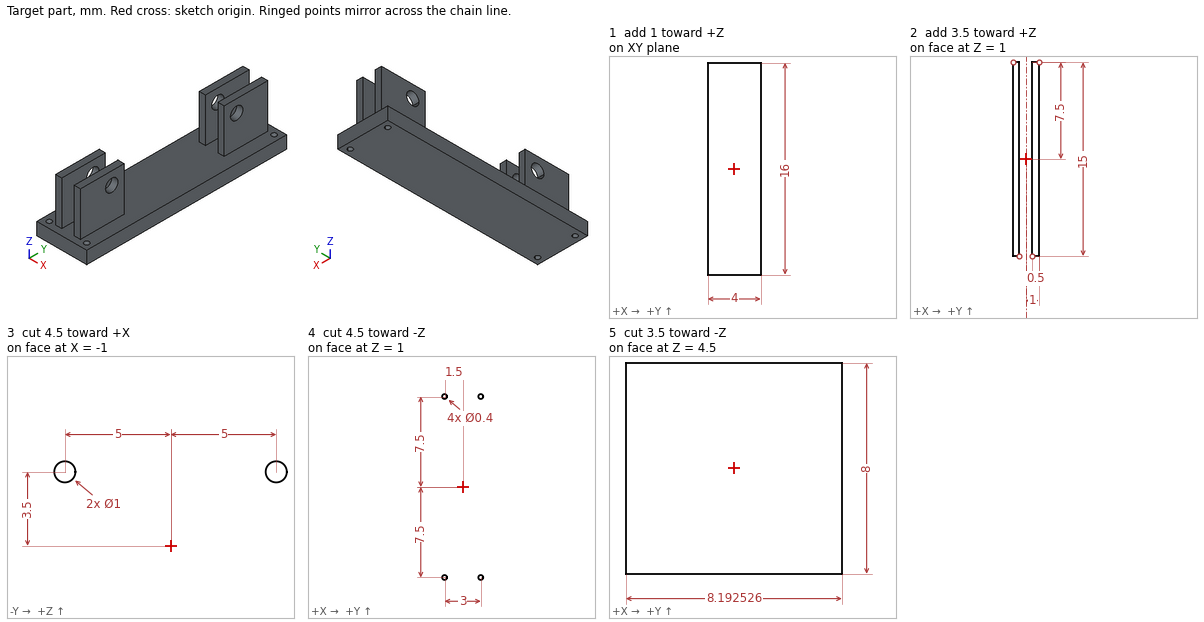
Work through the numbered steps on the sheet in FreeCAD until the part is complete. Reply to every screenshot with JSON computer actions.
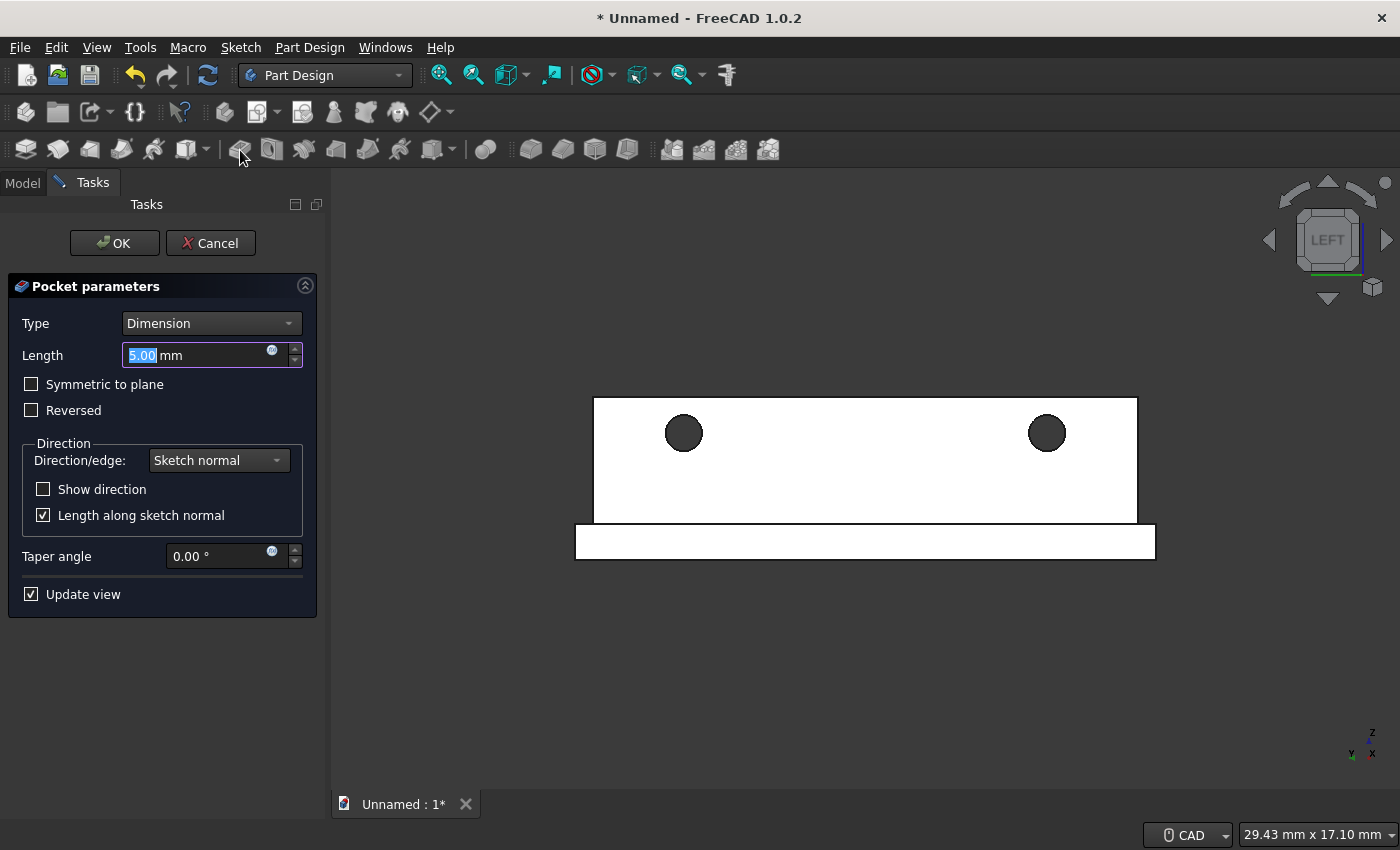
{"action": "type", "text": "4.5"}
{"action": "key", "text": "Tab"}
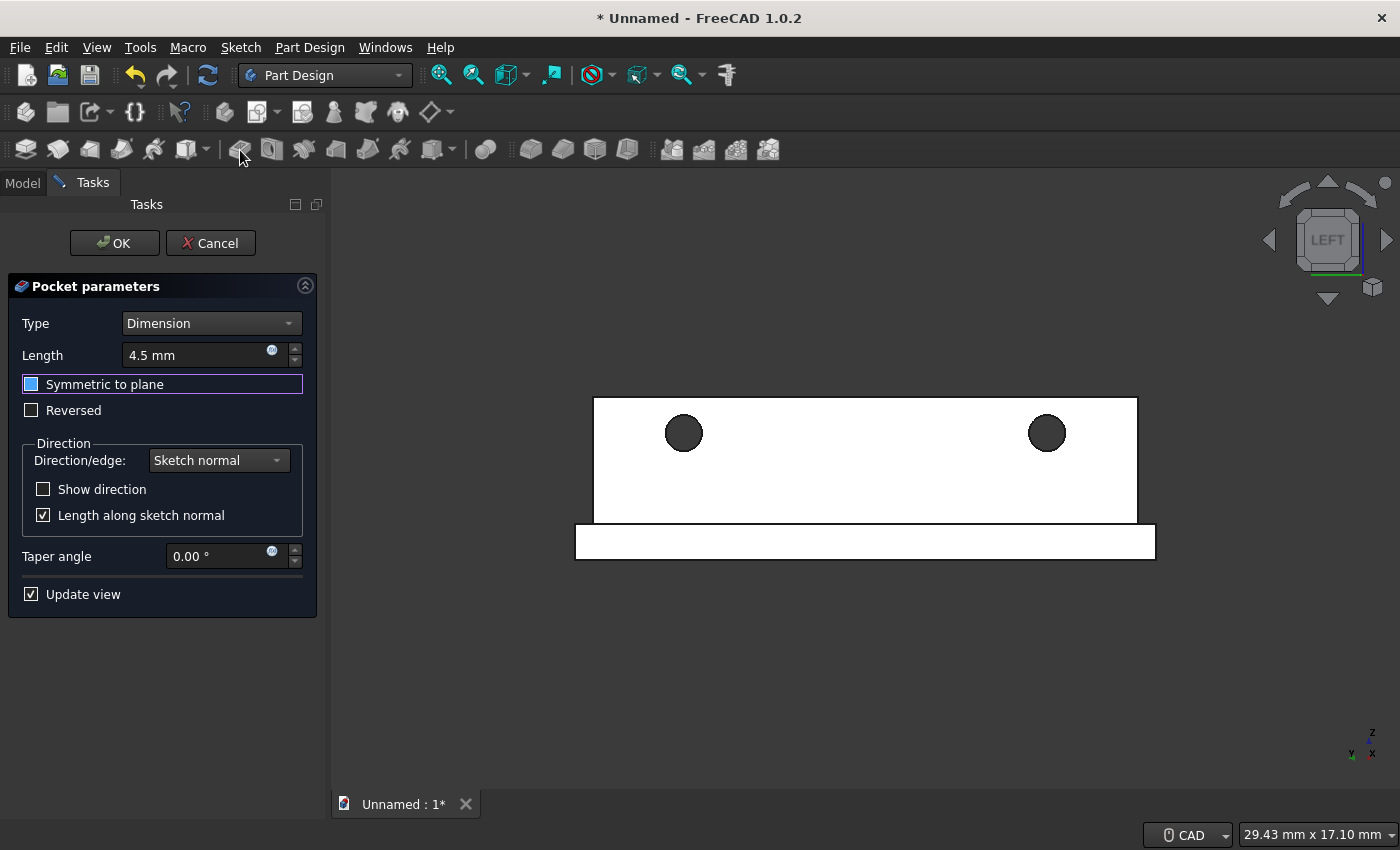
{"action": "left_click", "coordinate": [115, 243]}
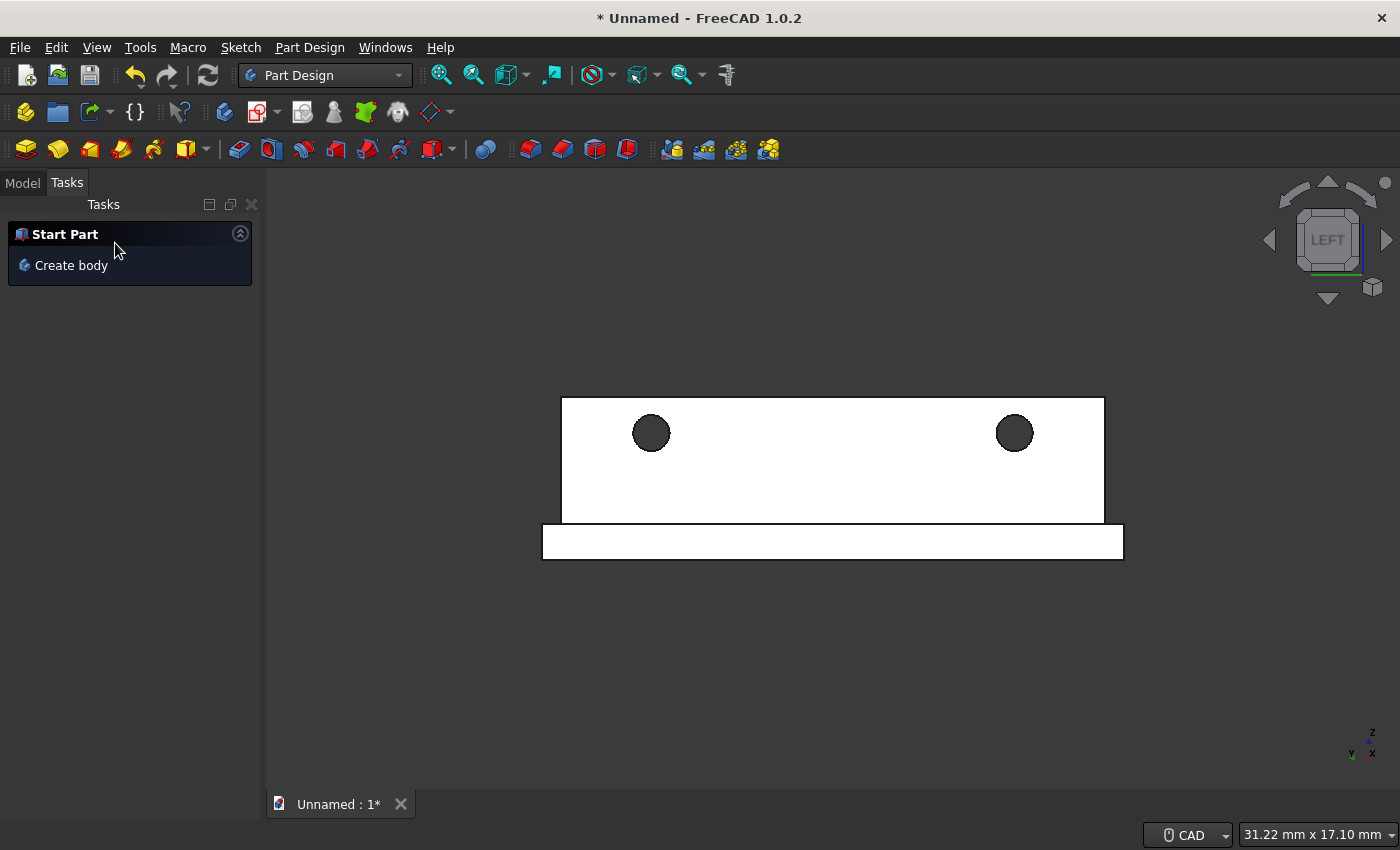
{"action": "key", "text": "0"}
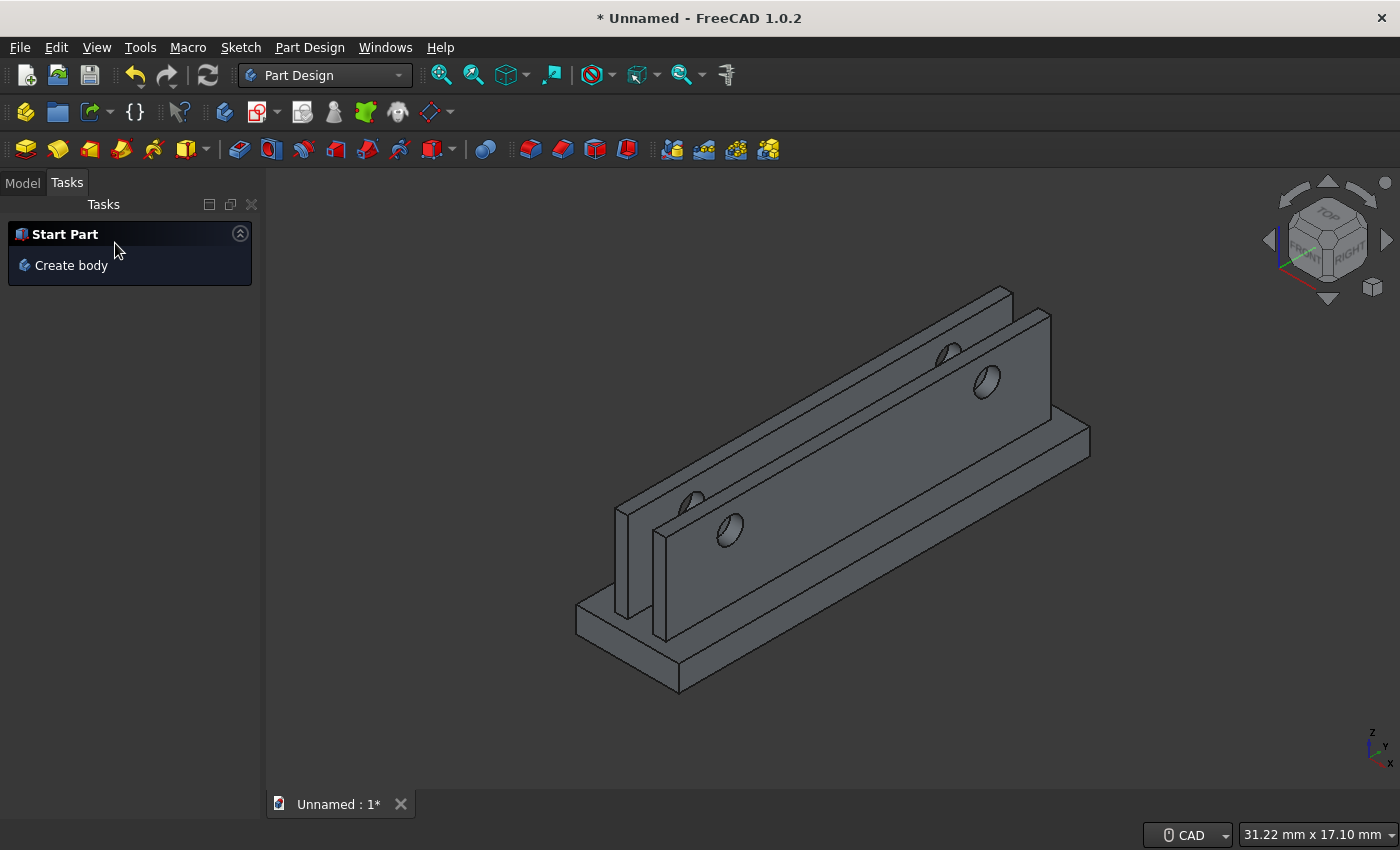
{"action": "key", "text": "2"}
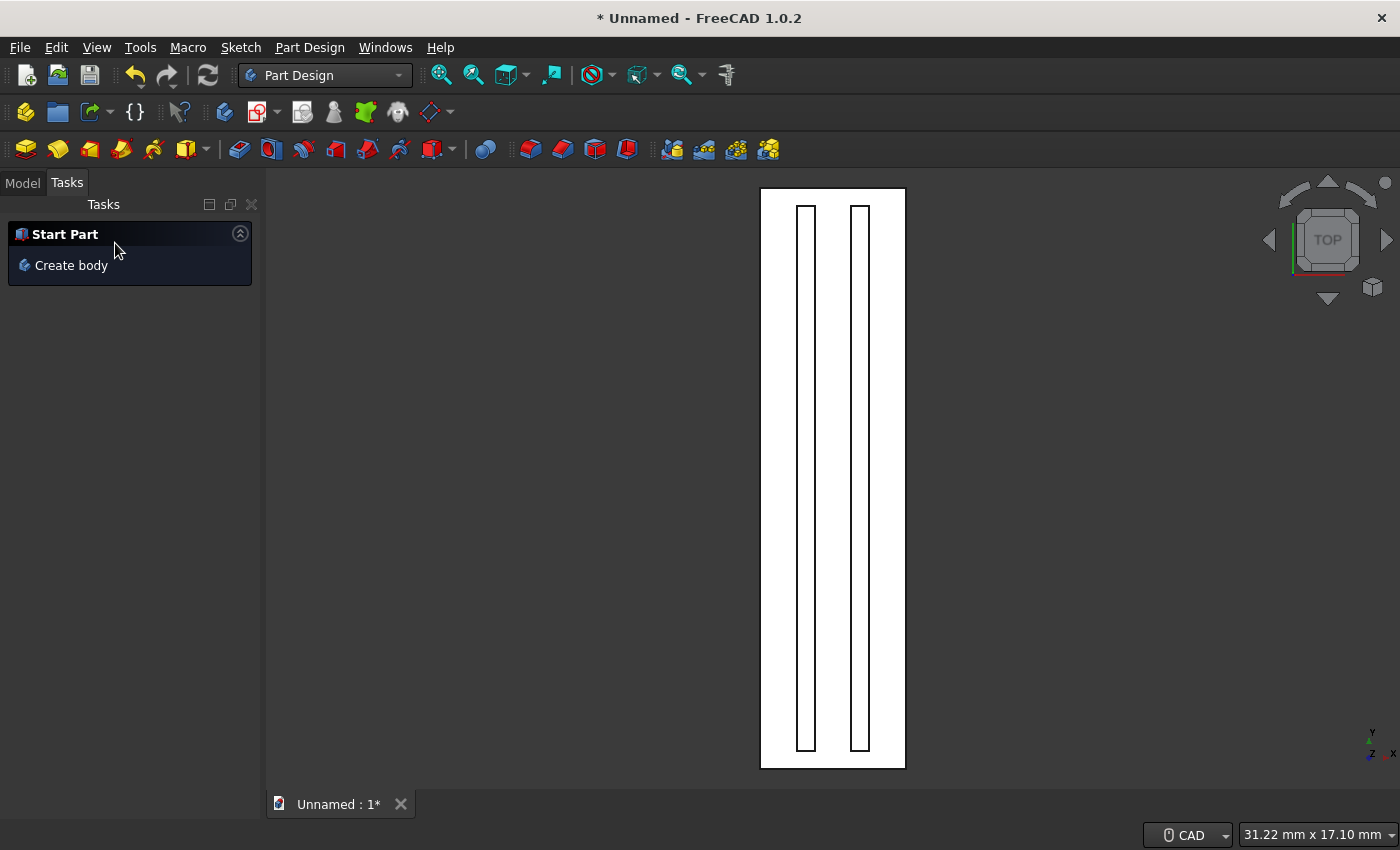
{"action": "left_click", "coordinate": [833, 228]}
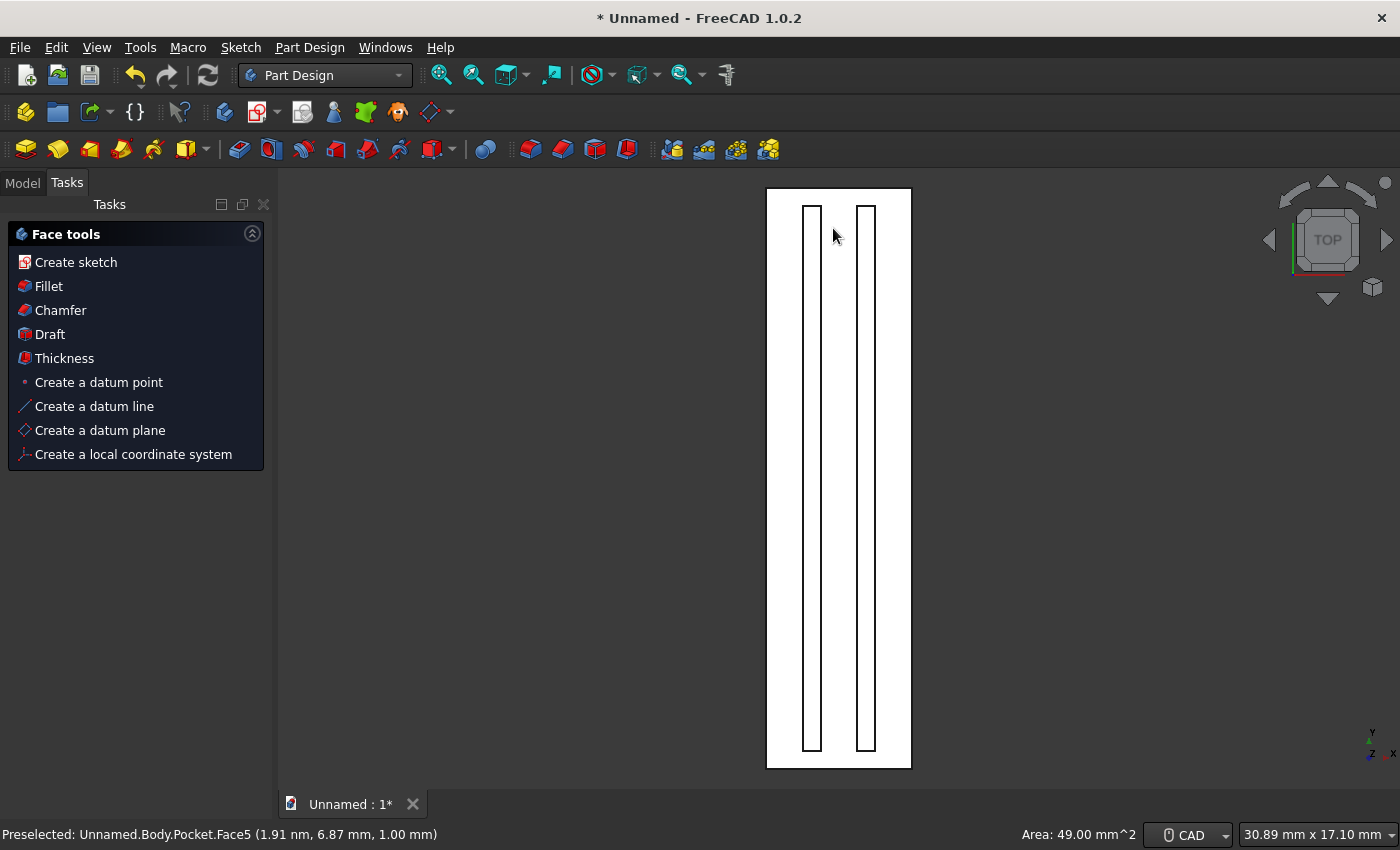
{"action": "left_click", "coordinate": [258, 112]}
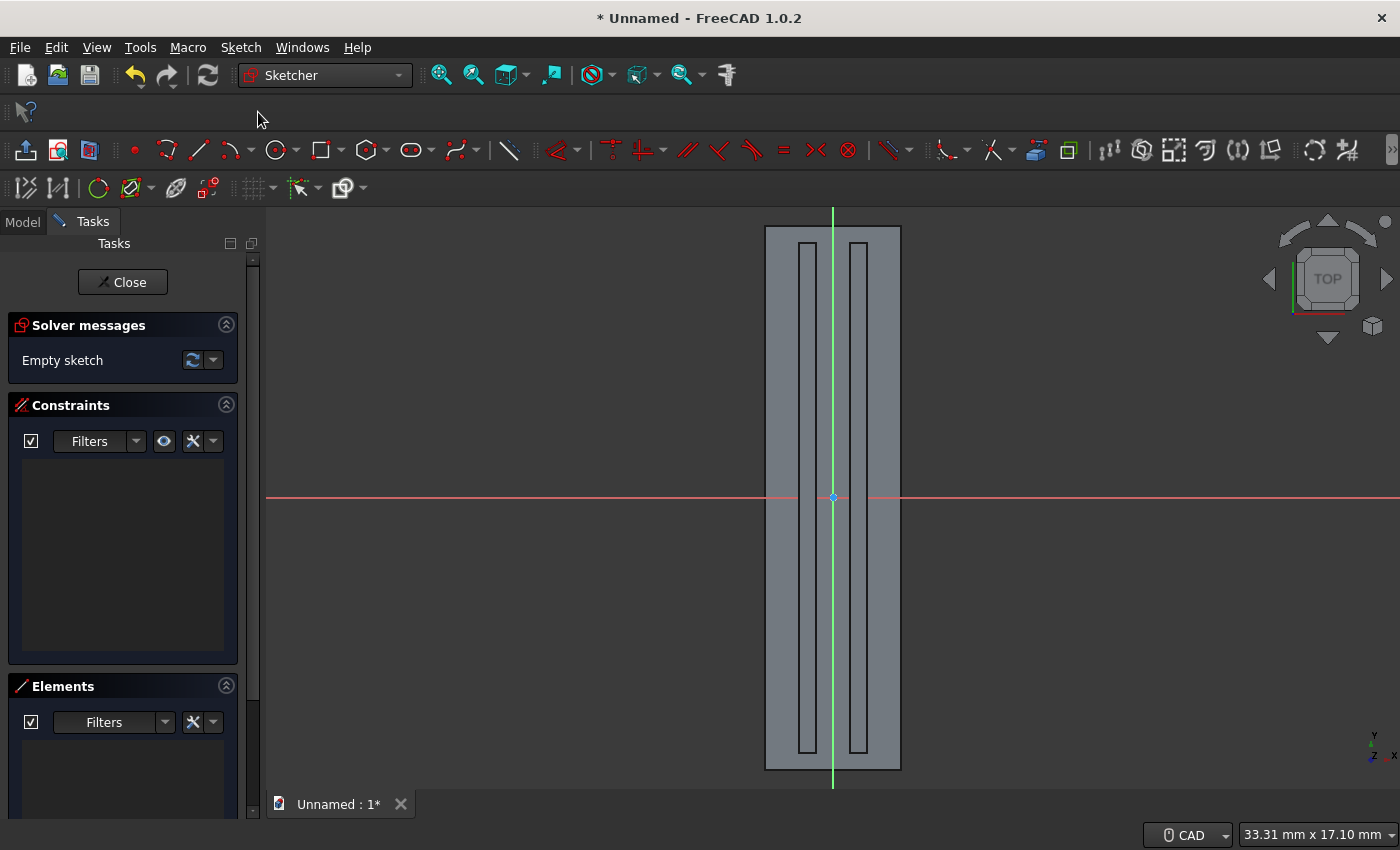
{"action": "scroll", "coordinate": [625, 498], "scroll_direction": "down", "scroll_amount": 2}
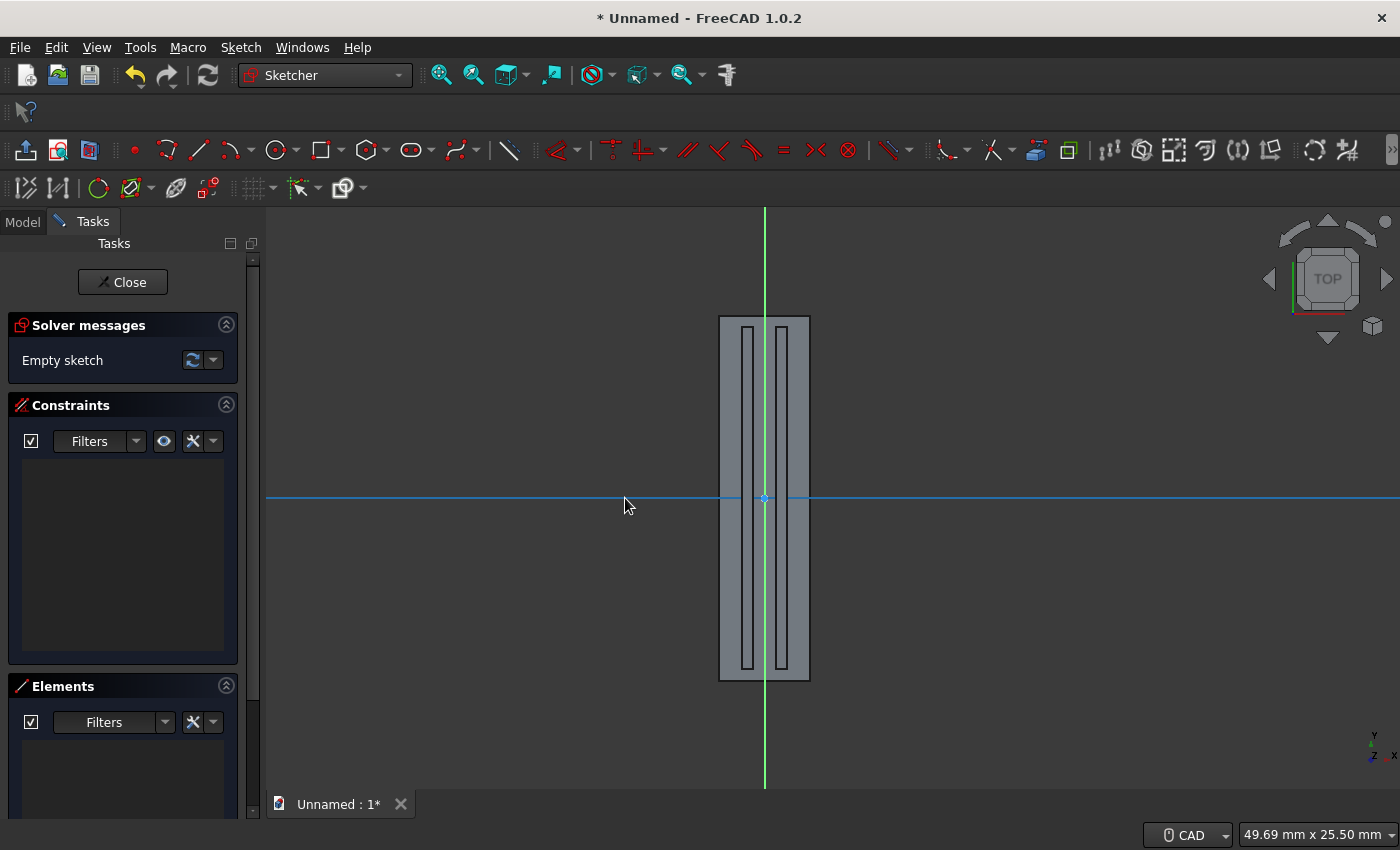
{"action": "key", "text": "g c"}